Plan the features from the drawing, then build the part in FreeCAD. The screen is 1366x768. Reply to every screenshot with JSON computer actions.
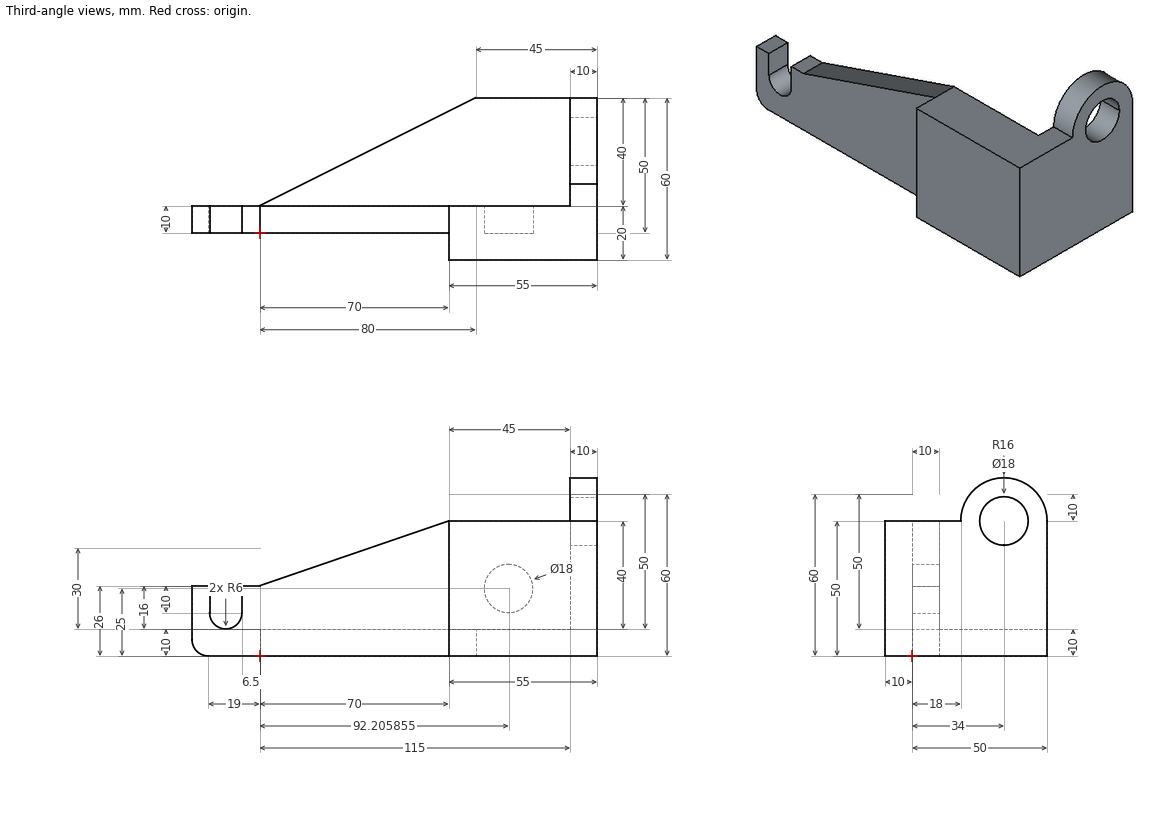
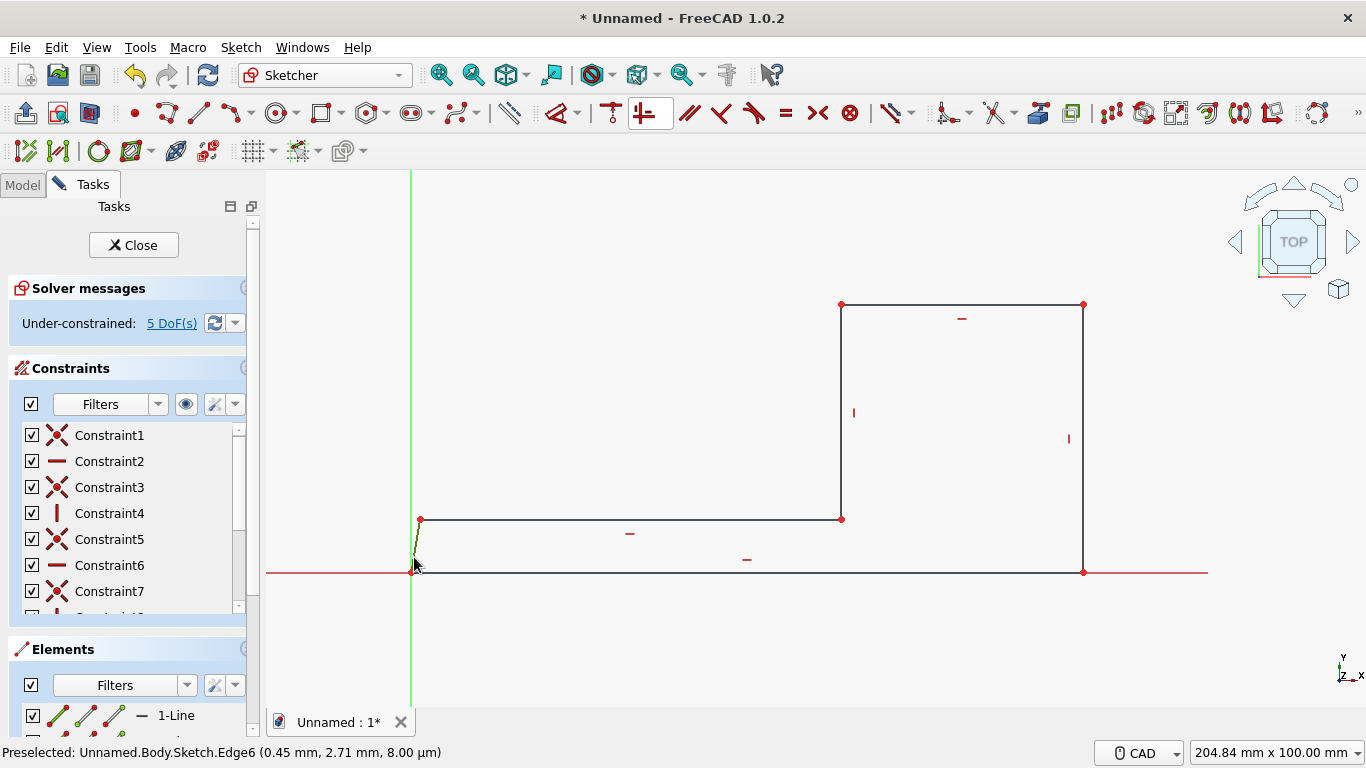
{"action": "key", "text": "v"}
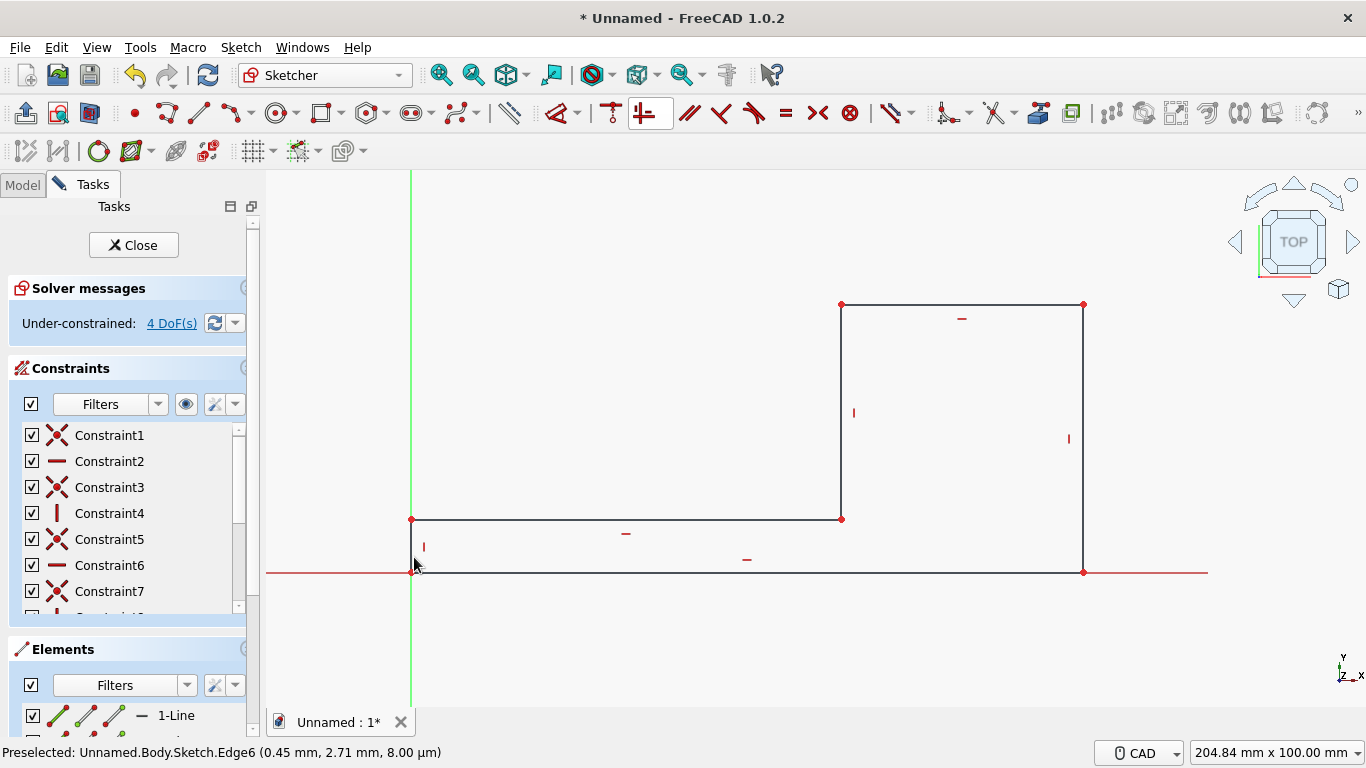
{"action": "left_click", "coordinate": [556, 114]}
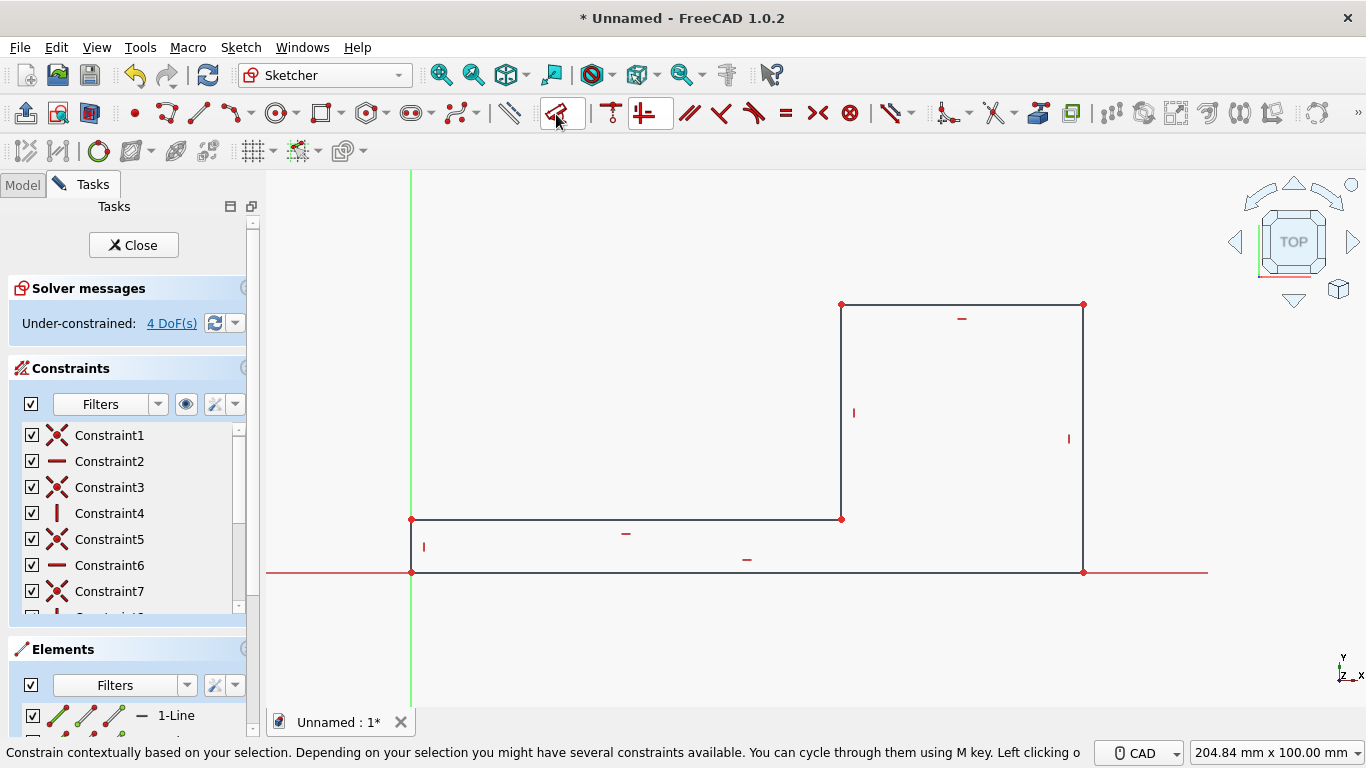
{"action": "left_click", "coordinate": [1083, 492]}
{"action": "left_click", "coordinate": [1117, 439]}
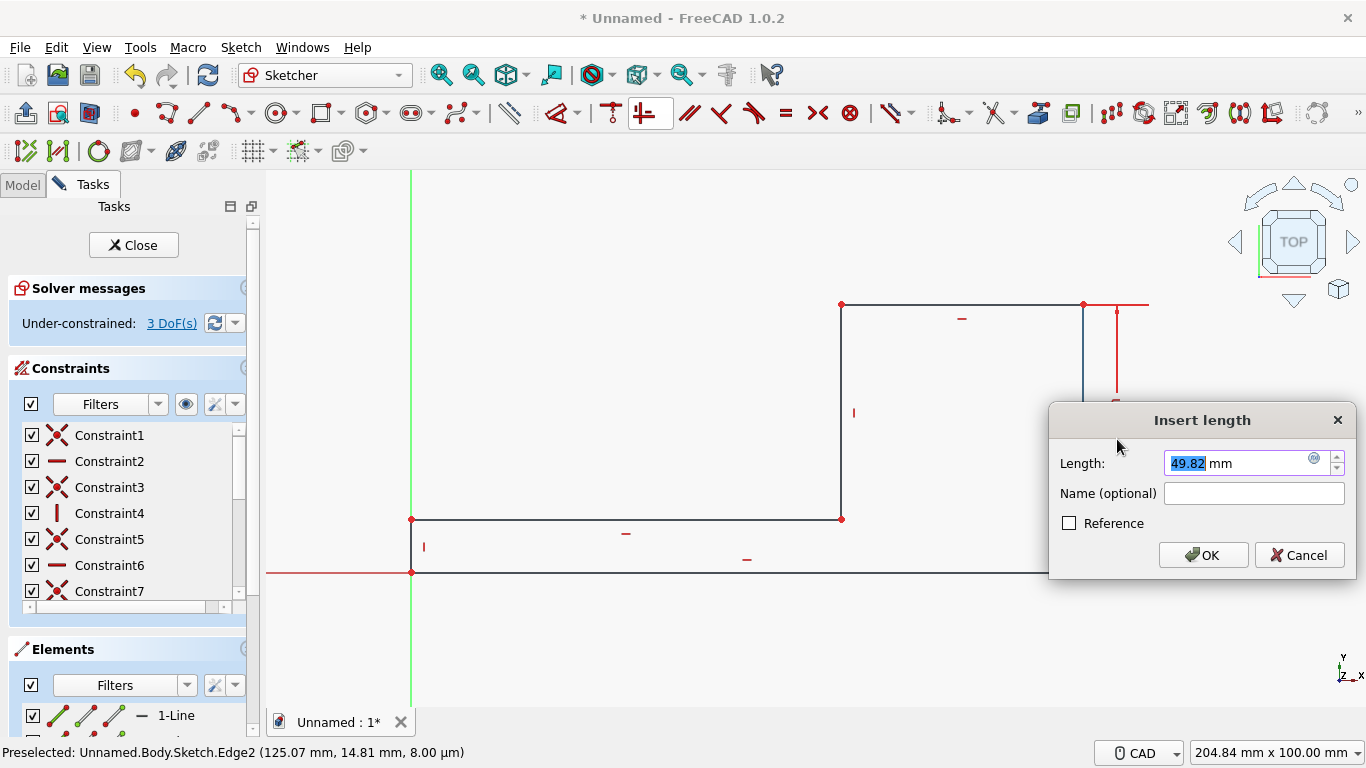
{"action": "type", "text": "50"}
{"action": "key", "text": "Return"}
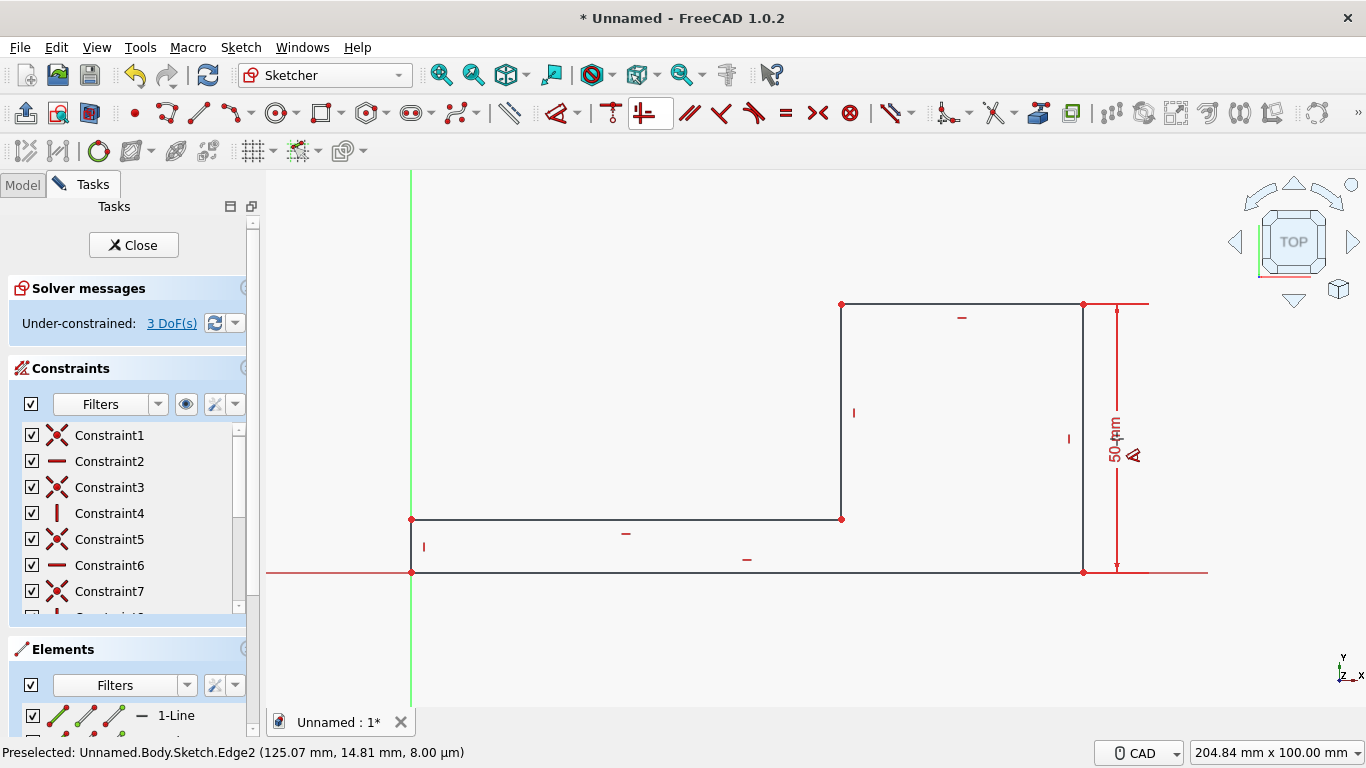
{"action": "left_click", "coordinate": [1010, 304]}
{"action": "left_click", "coordinate": [962, 270]}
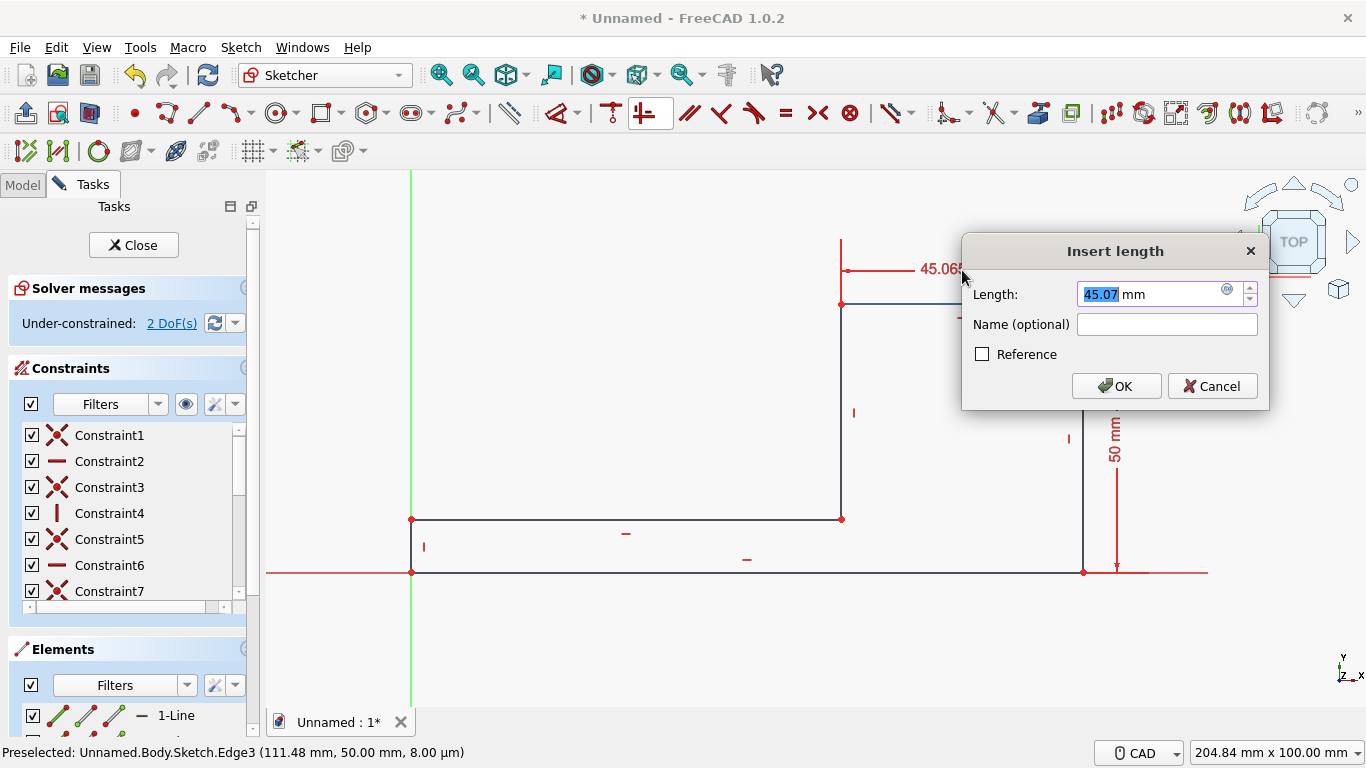
{"action": "type", "text": "45"}
{"action": "key", "text": "Return"}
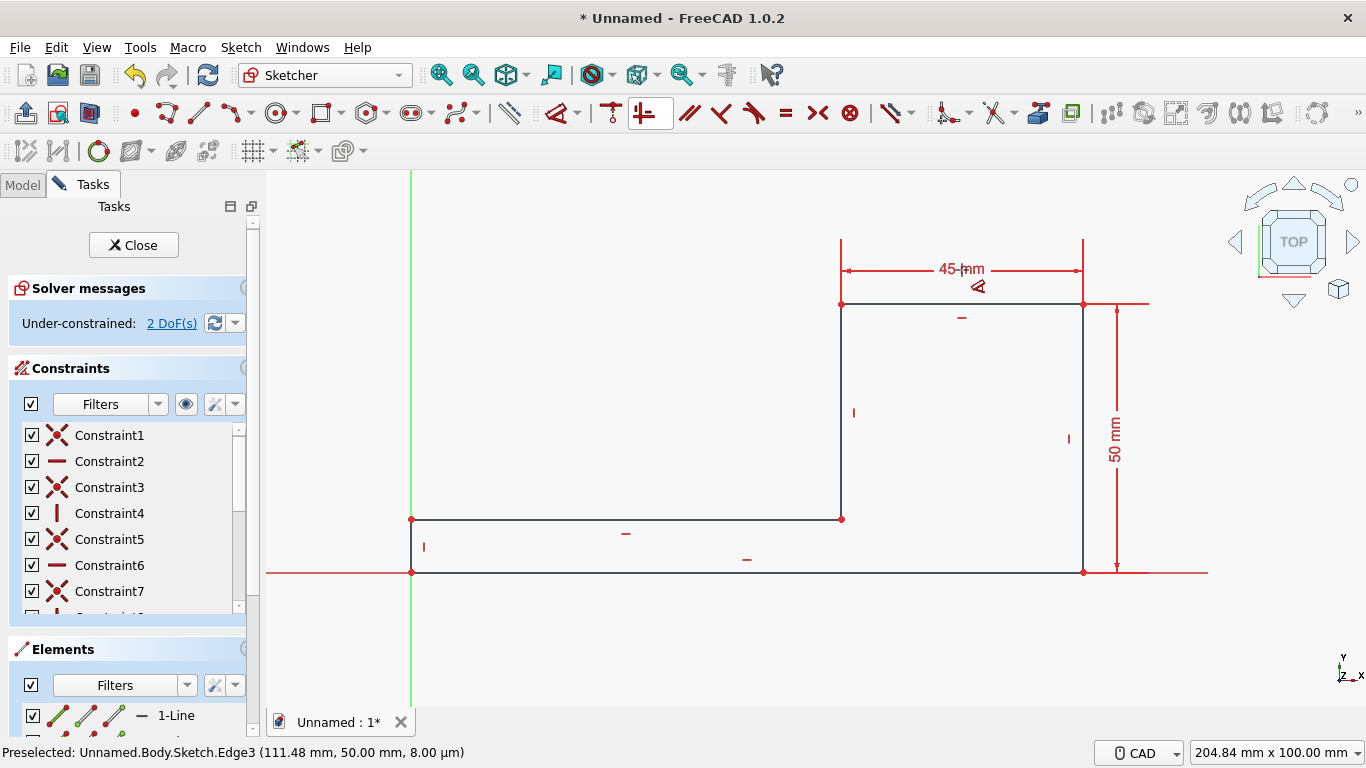
{"action": "left_click", "coordinate": [841, 369]}
{"action": "left_click", "coordinate": [875, 412]}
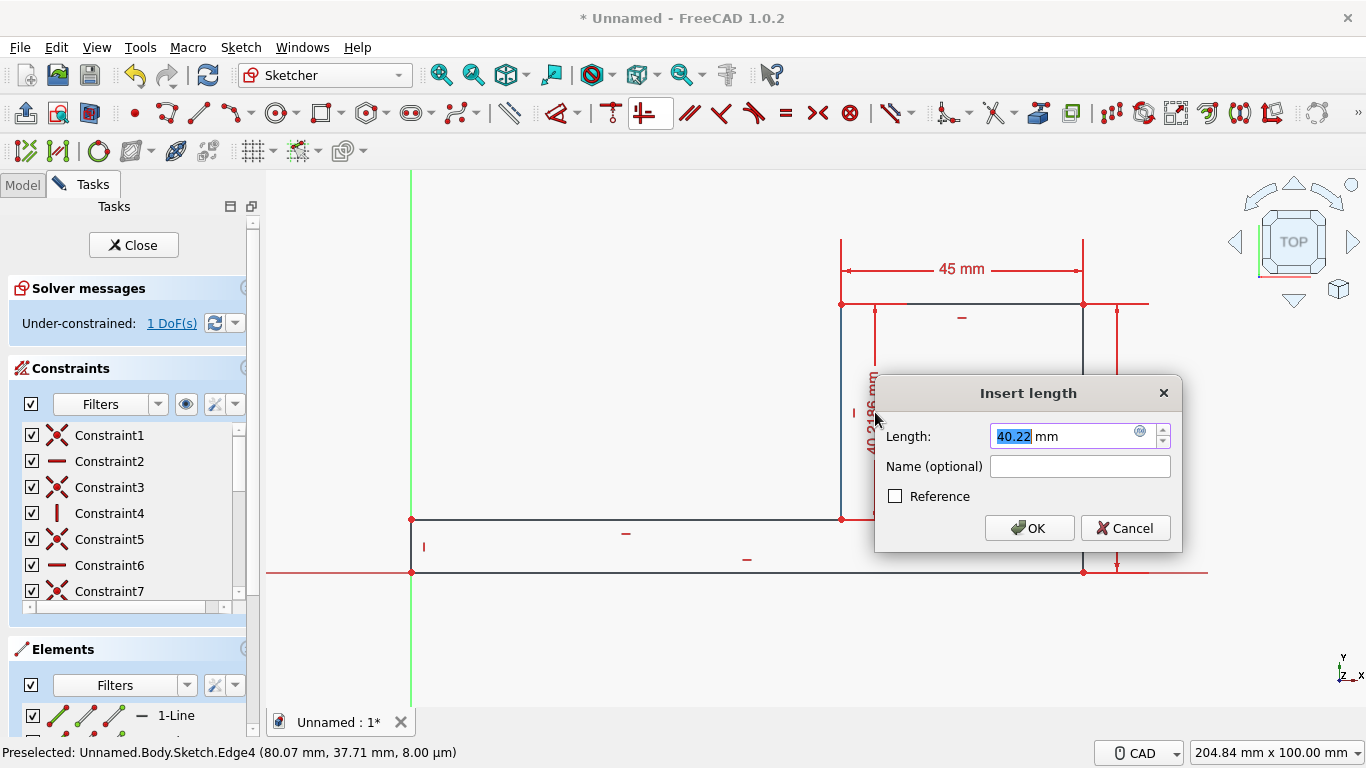
{"action": "type", "text": "40"}
{"action": "key", "text": "Return"}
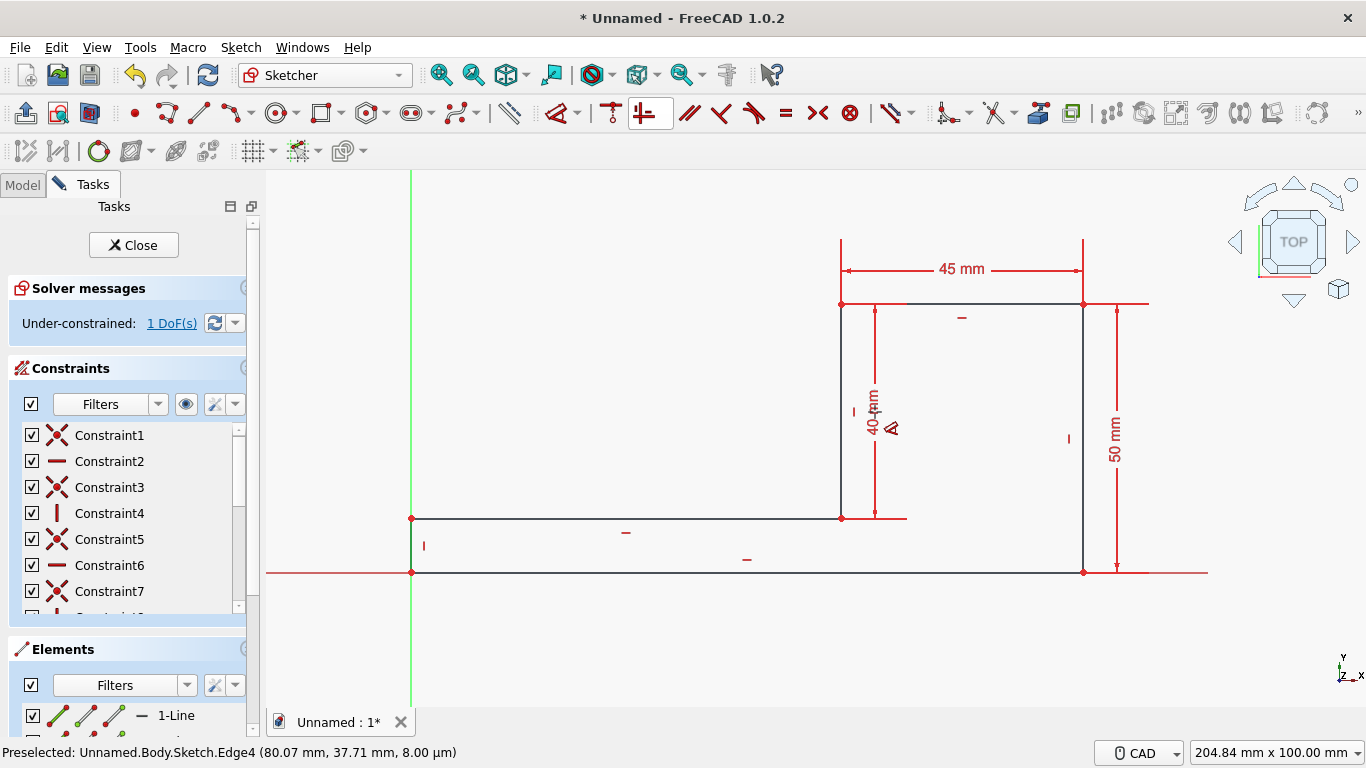
{"action": "left_click", "coordinate": [712, 519]}
{"action": "left_click", "coordinate": [626, 553]}